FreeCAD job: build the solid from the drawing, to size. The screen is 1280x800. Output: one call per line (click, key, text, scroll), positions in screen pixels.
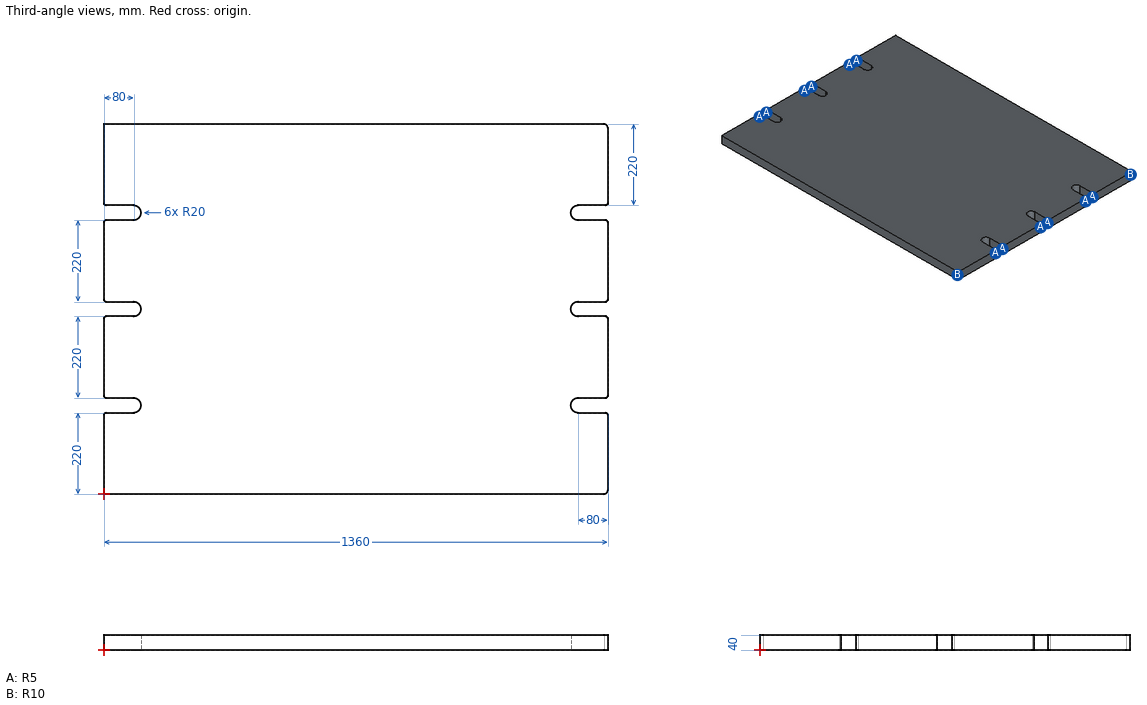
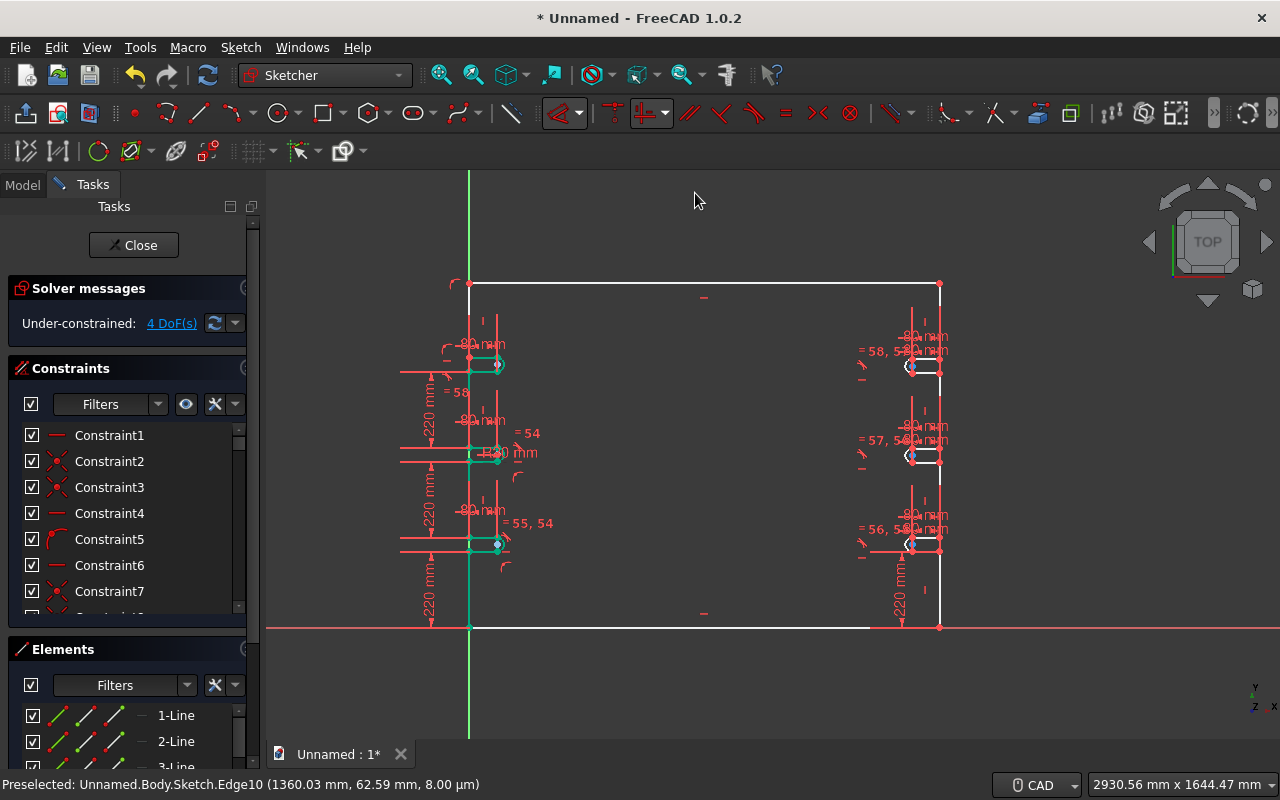
click(940, 485)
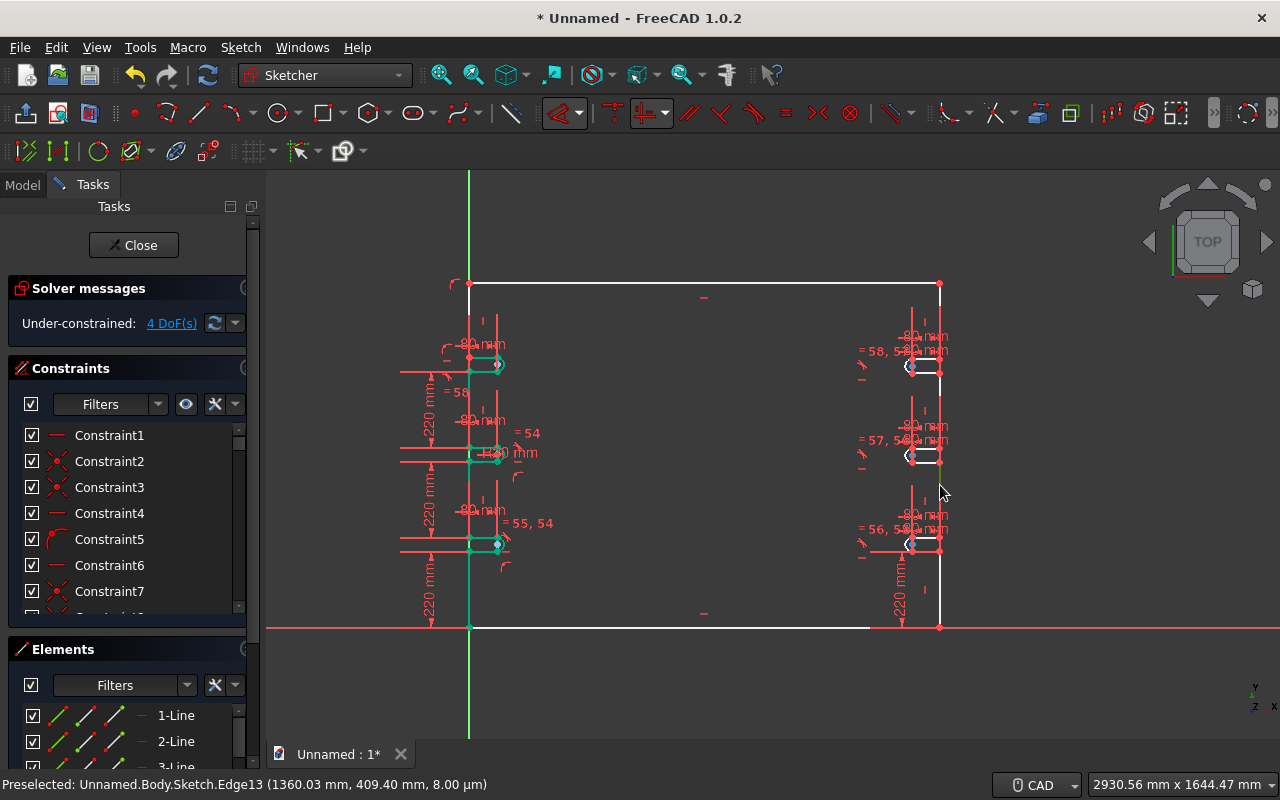
click(582, 114)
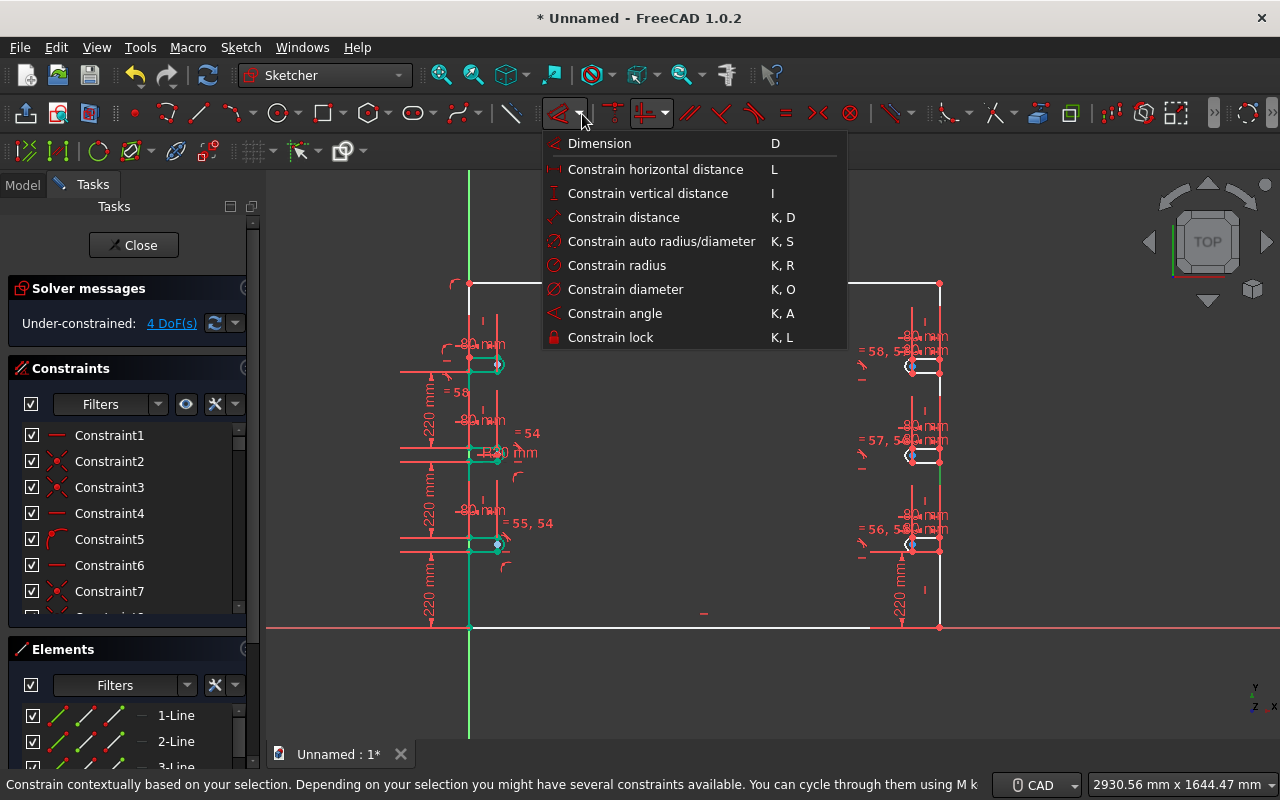
click(695, 193)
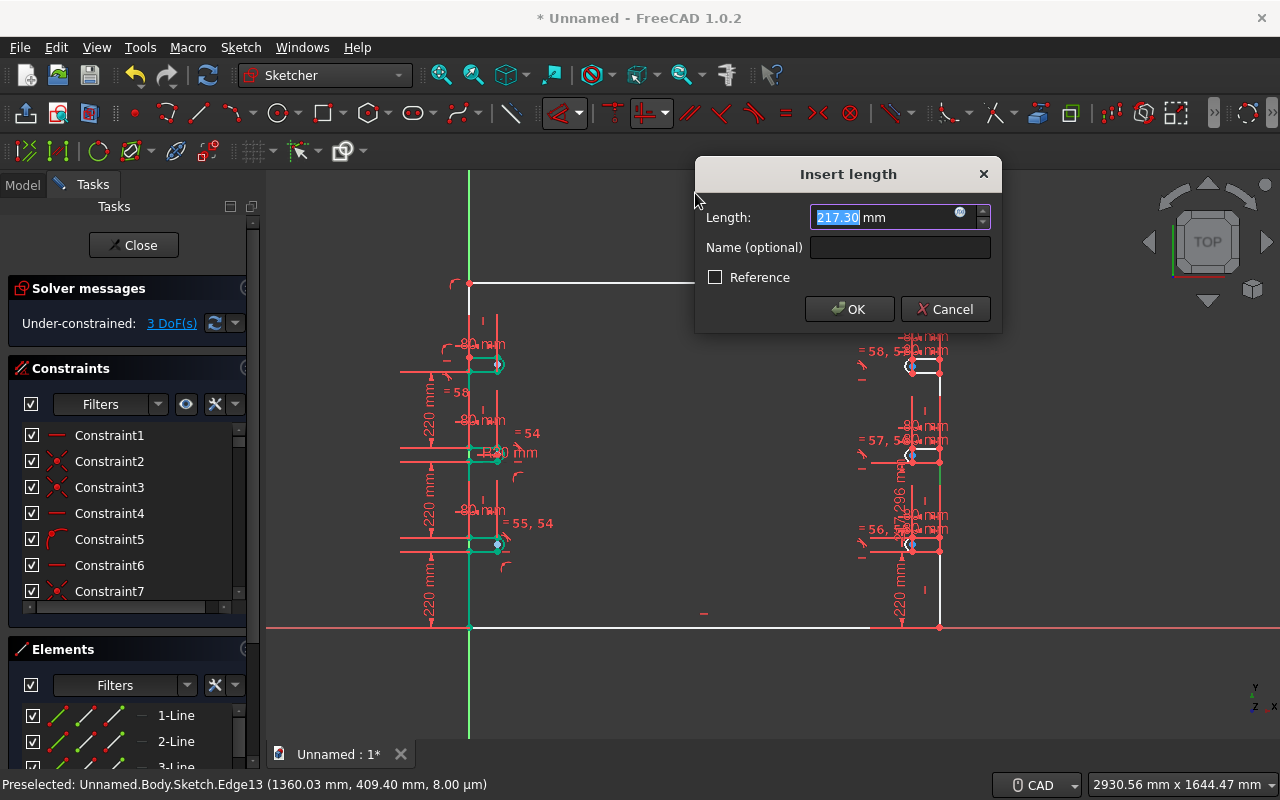
text(220)
key(Return)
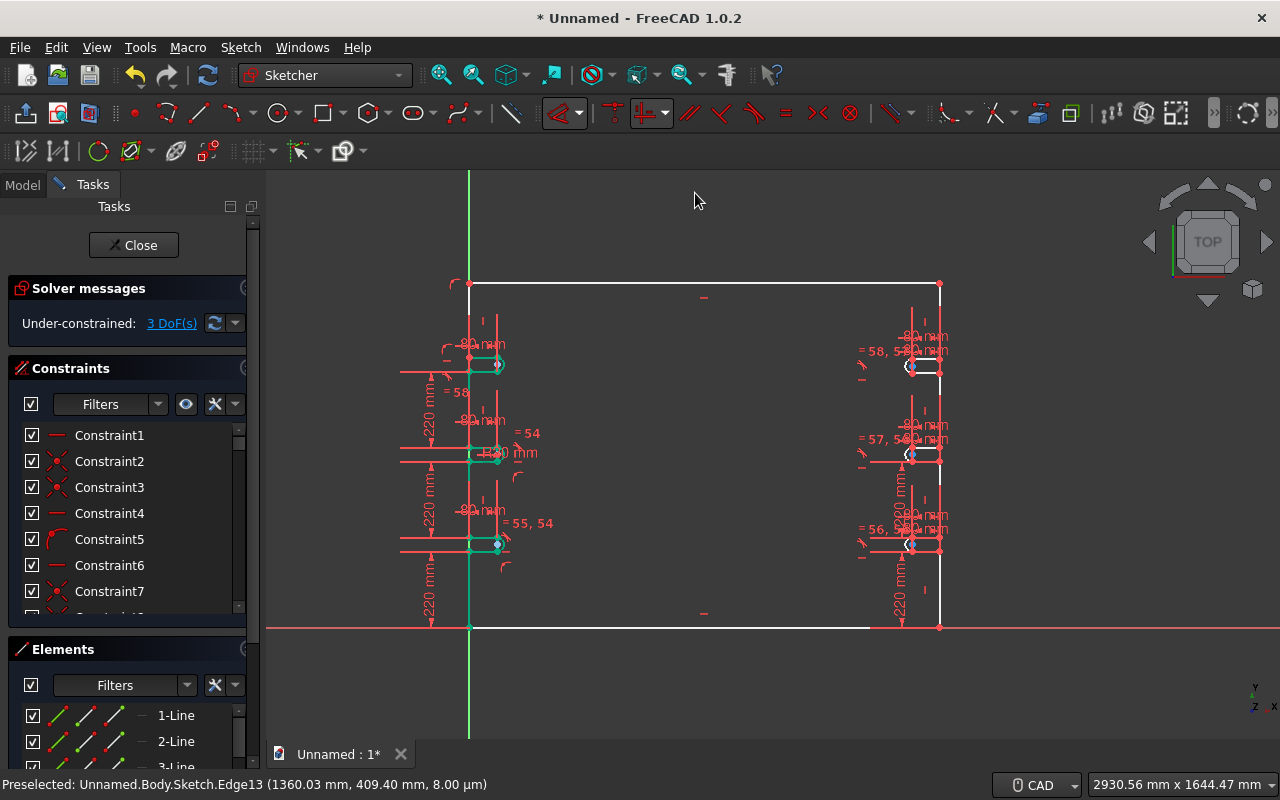
click(940, 395)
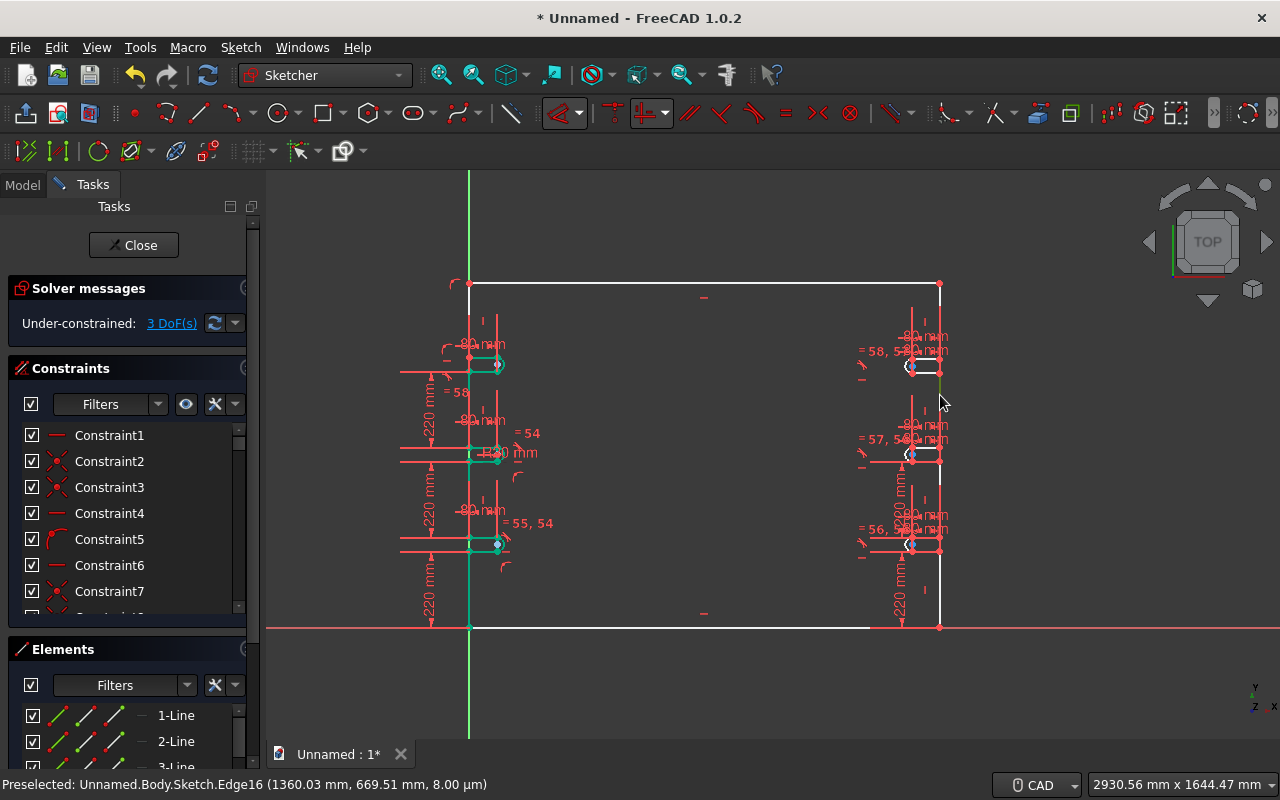
click(582, 114)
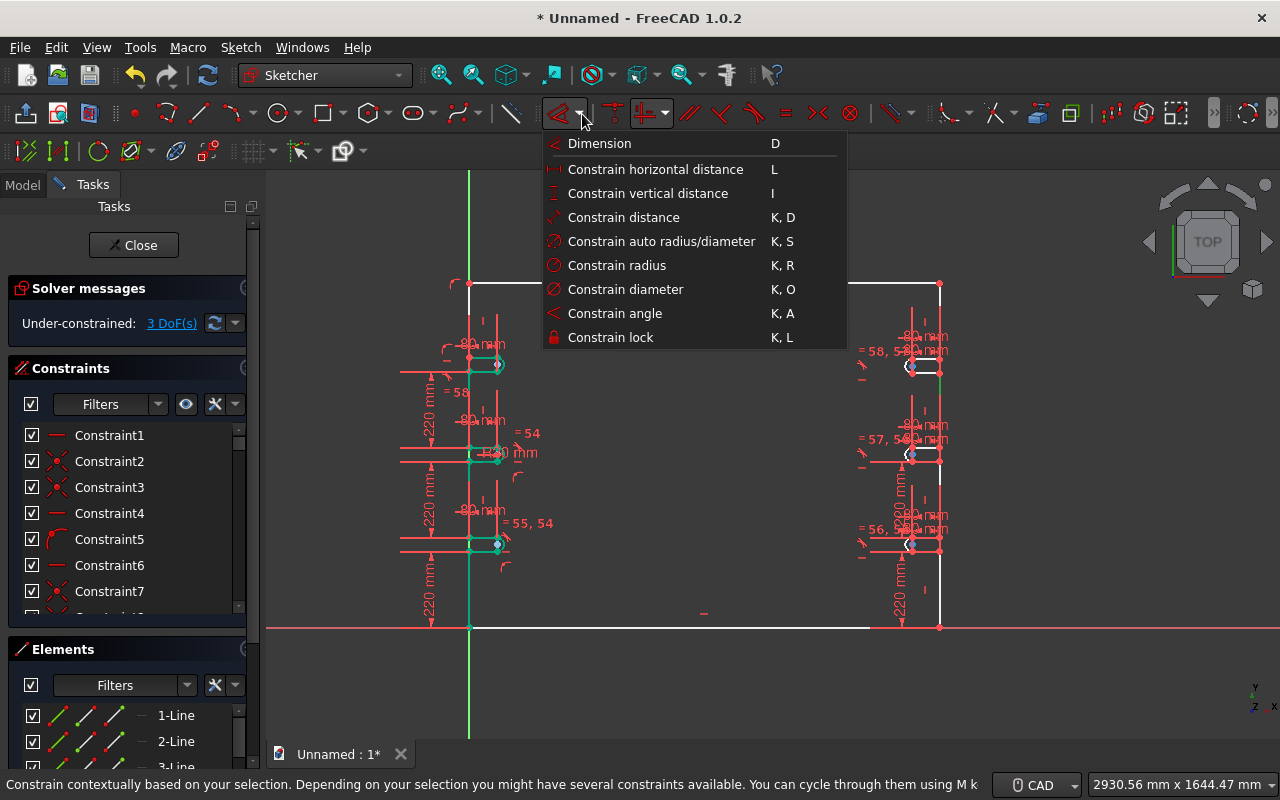
click(695, 193)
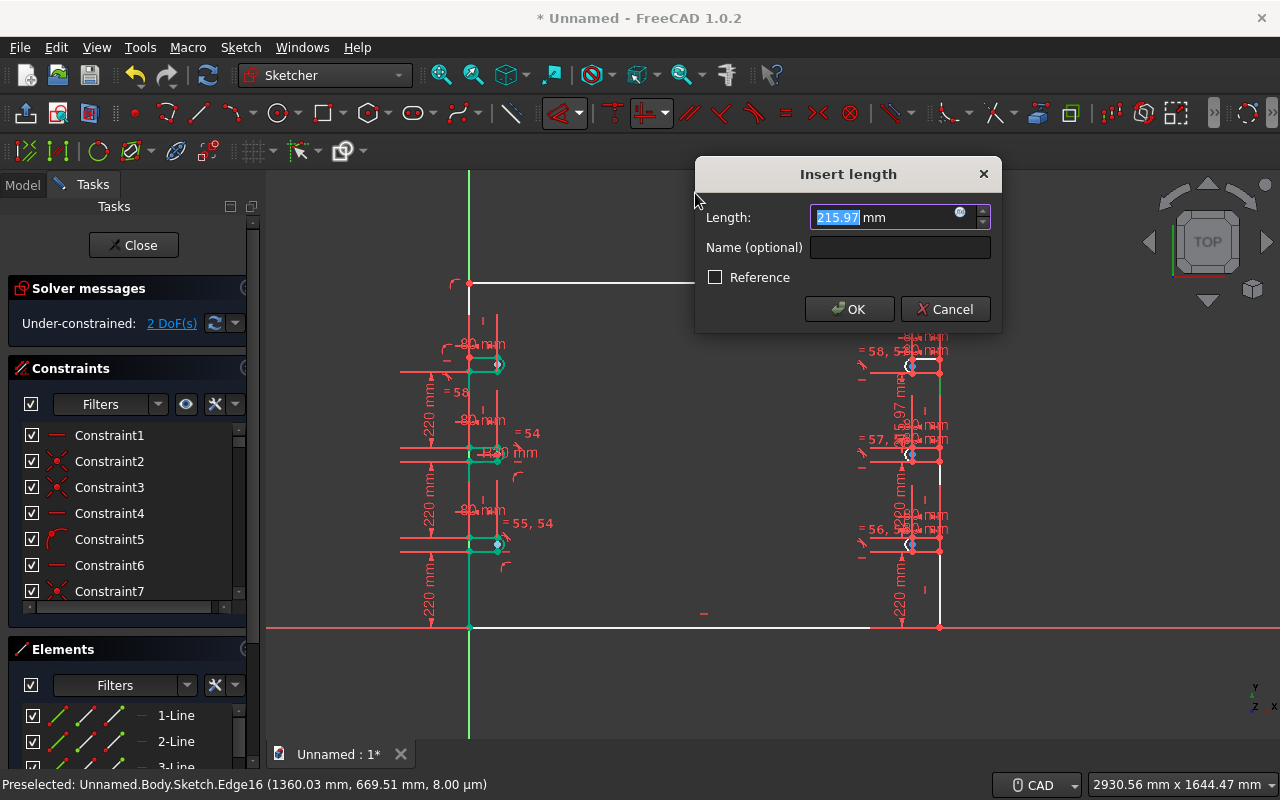
text(220)
key(Return)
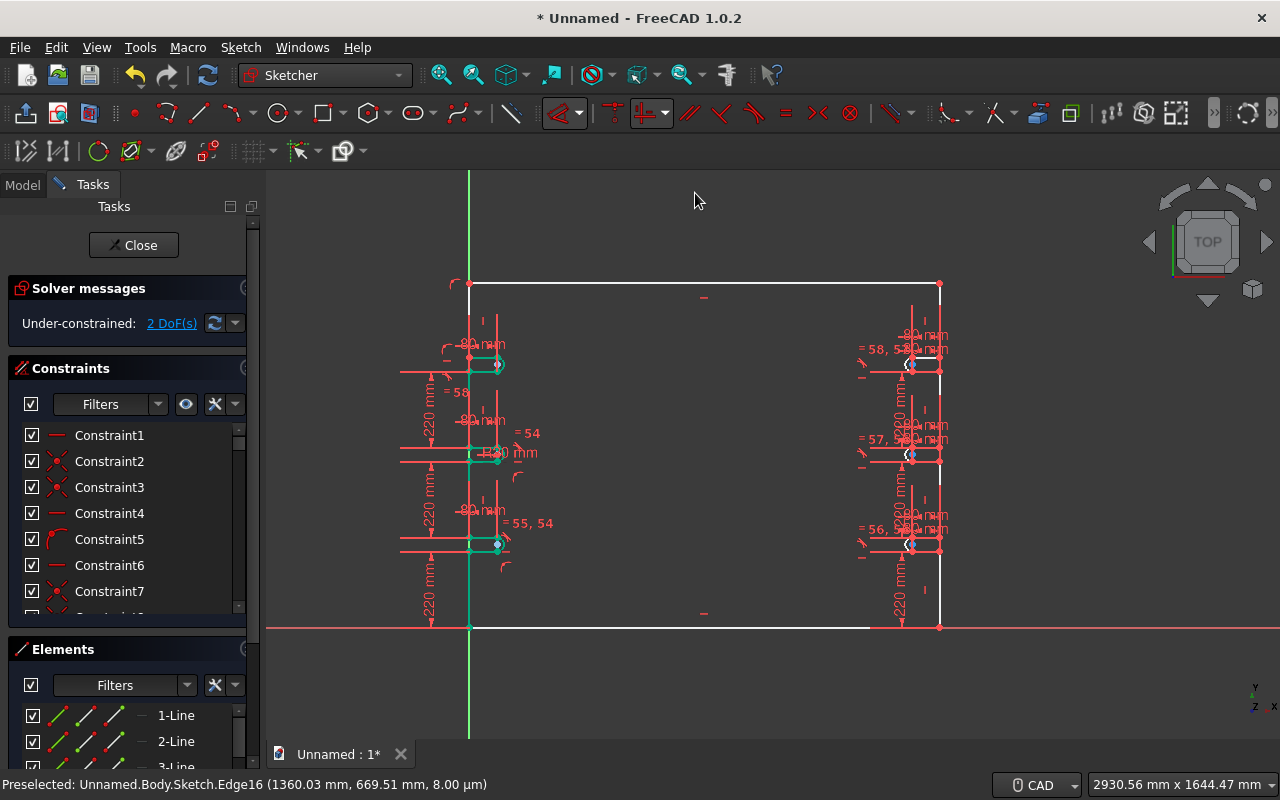
click(940, 306)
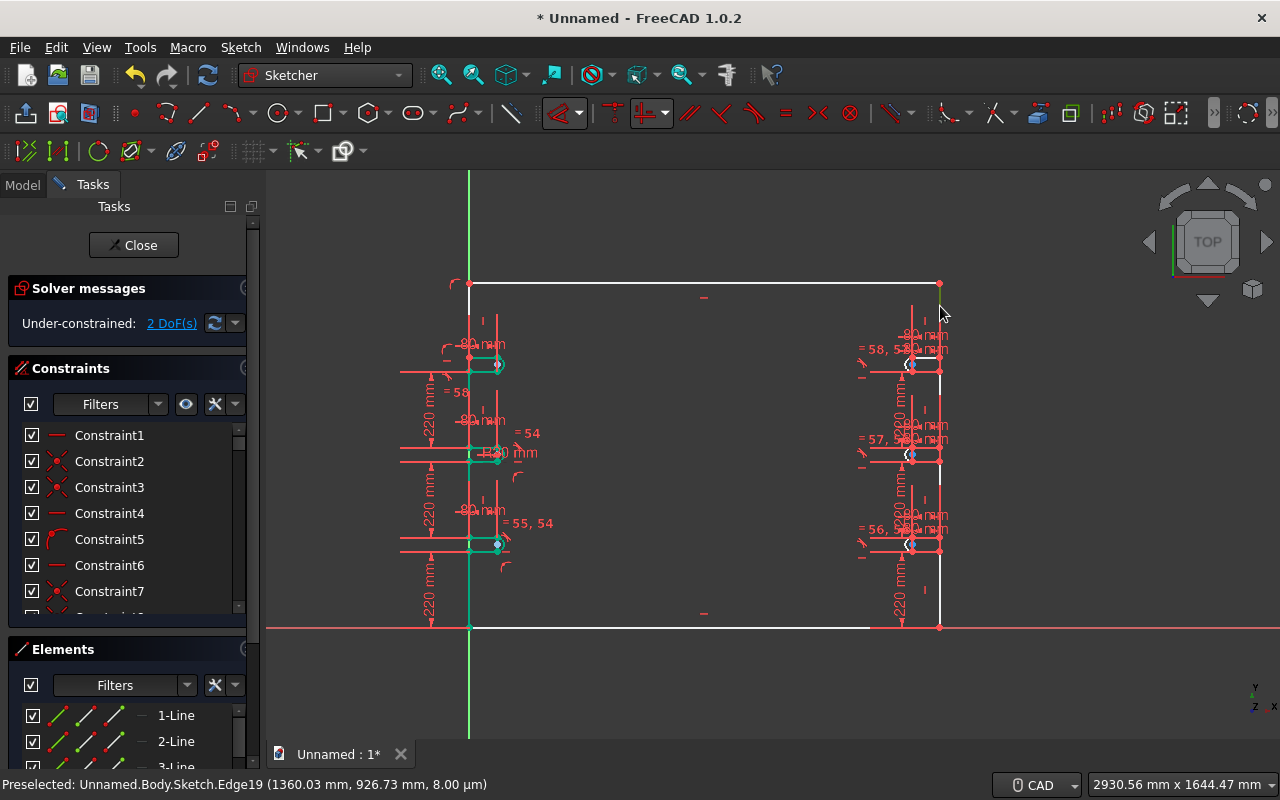
click(582, 114)